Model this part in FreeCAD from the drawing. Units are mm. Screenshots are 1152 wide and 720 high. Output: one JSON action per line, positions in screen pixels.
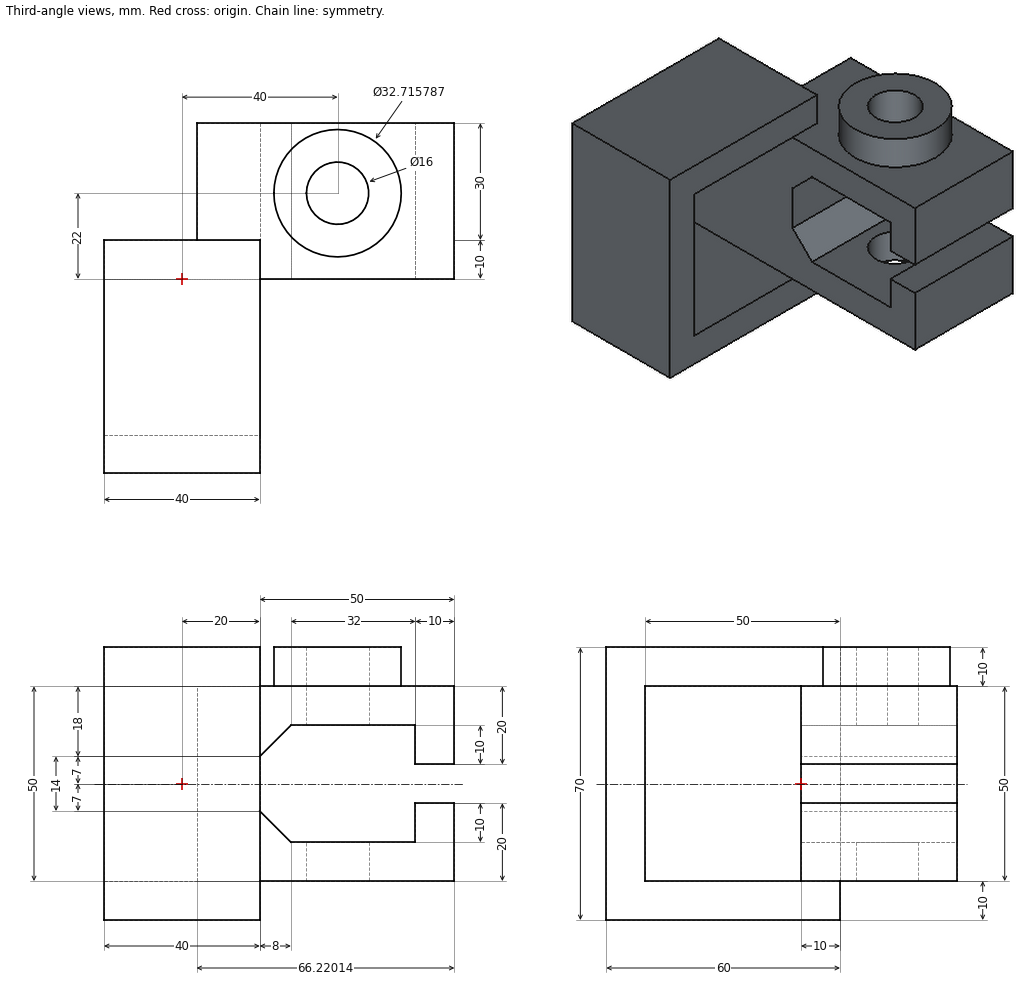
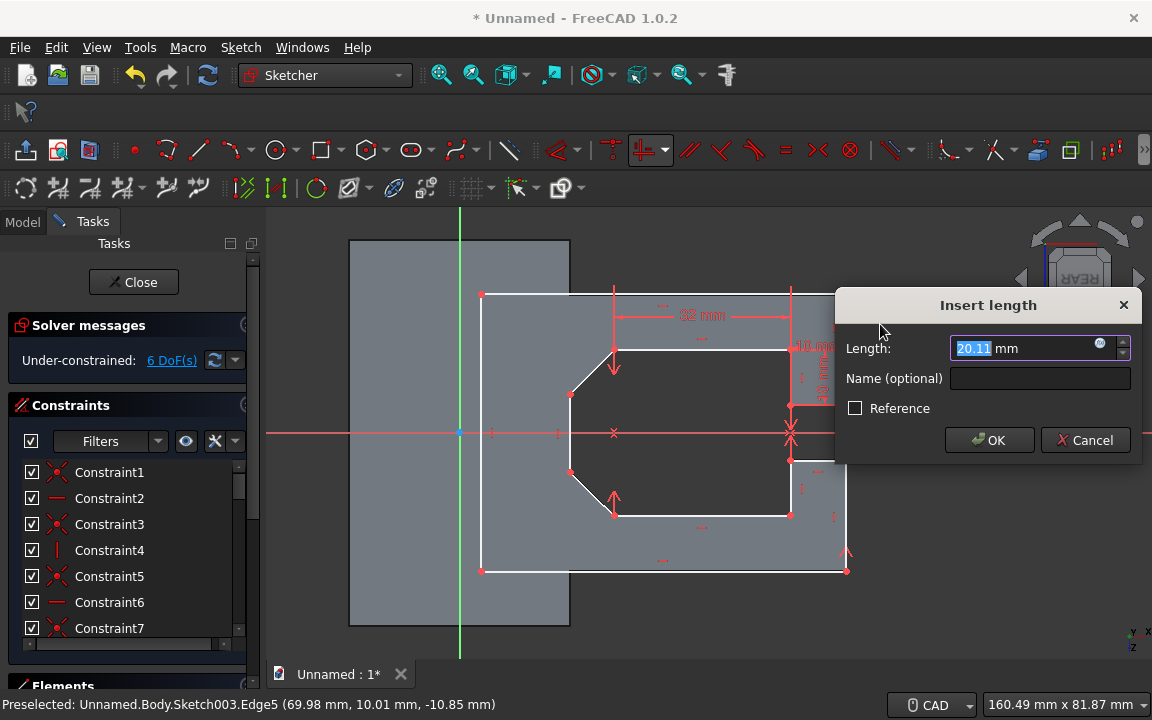
{"action": "type", "text": "20"}
{"action": "key", "text": "Return"}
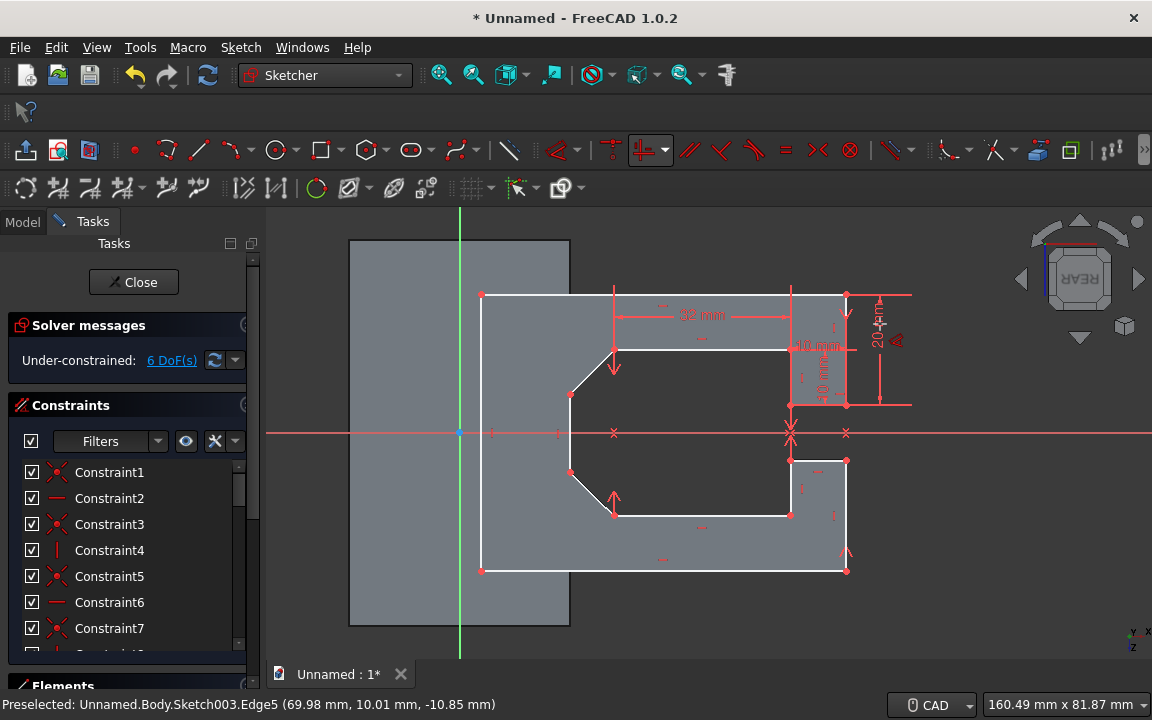
{"action": "left_click", "coordinate": [481, 378]}
{"action": "left_click", "coordinate": [515, 369]}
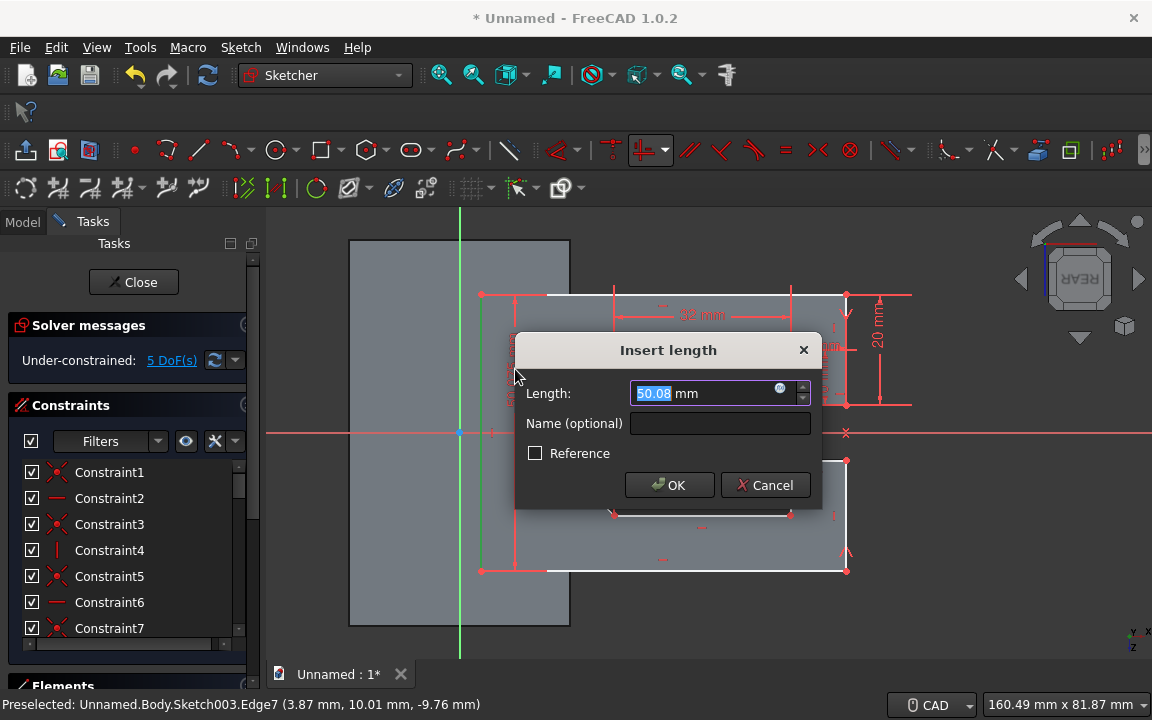
{"action": "type", "text": "50"}
{"action": "key", "text": "Return"}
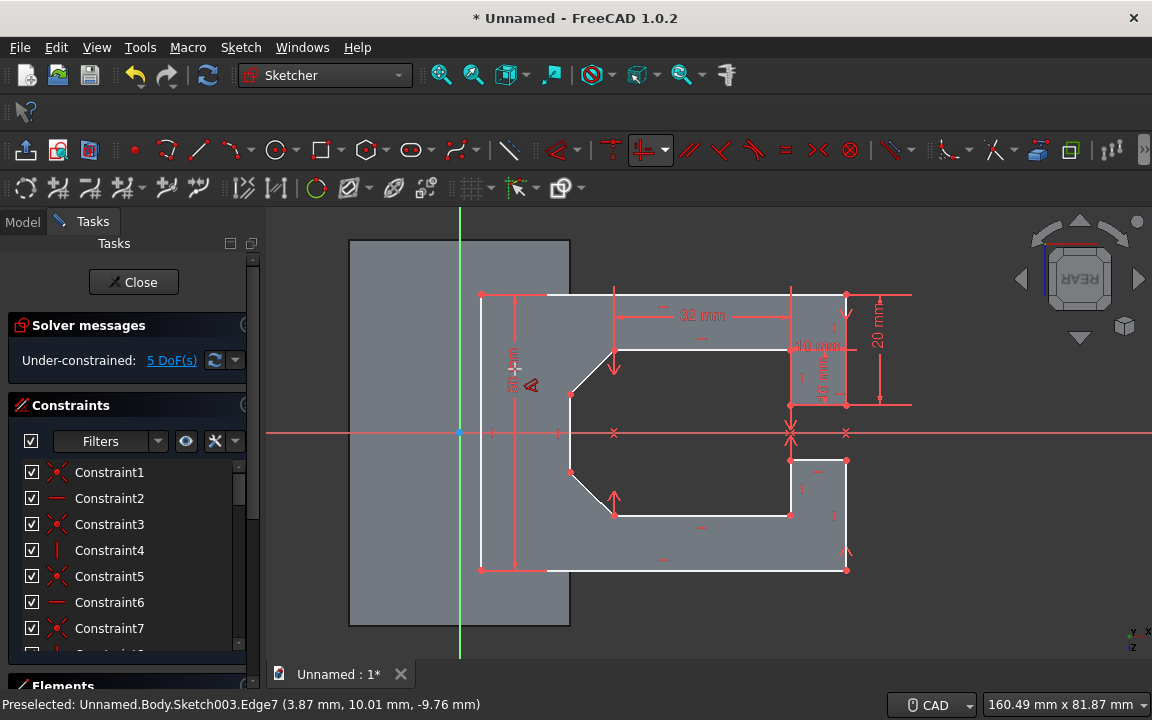
{"action": "left_click", "coordinate": [570, 450]}
{"action": "left_click", "coordinate": [536, 416]}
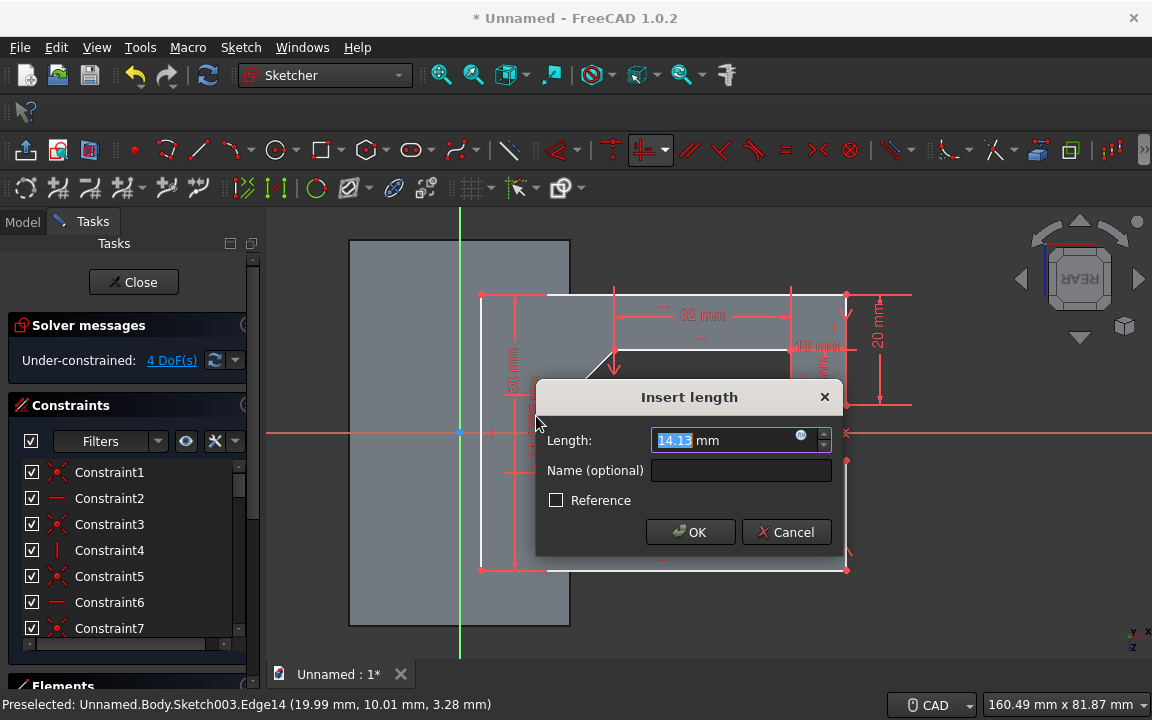
{"action": "type", "text": "14"}
{"action": "key", "text": "Return"}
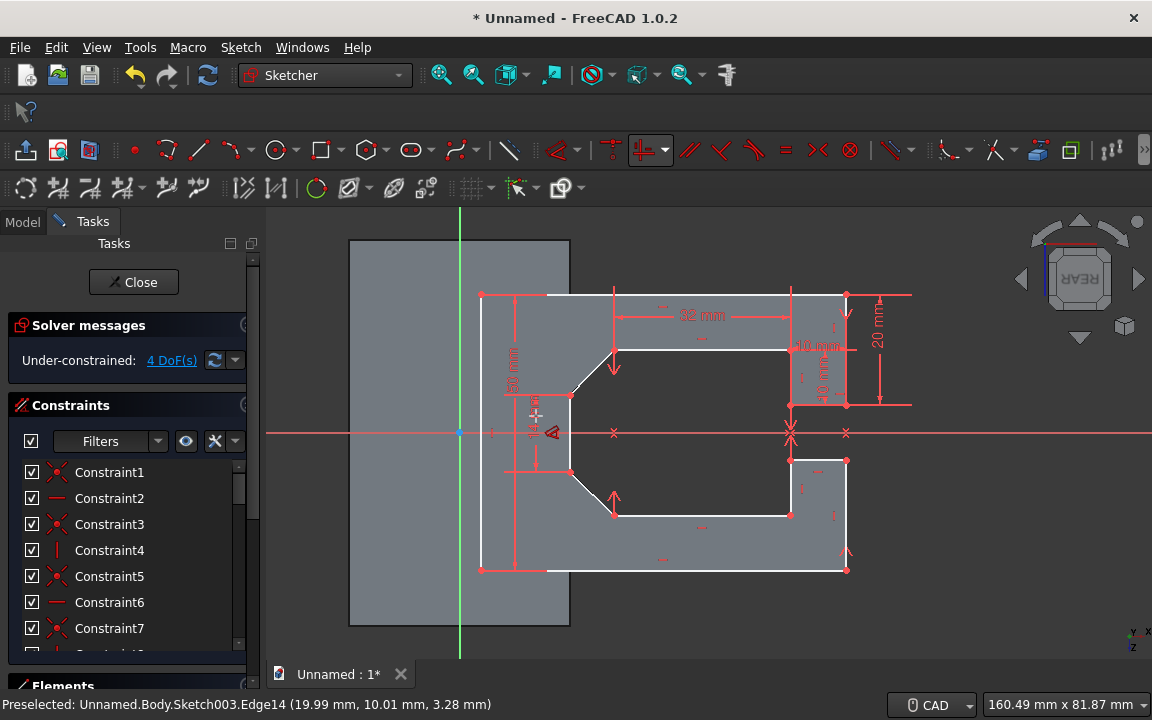
{"action": "left_click", "coordinate": [570, 395]}
{"action": "left_click", "coordinate": [426, 414]}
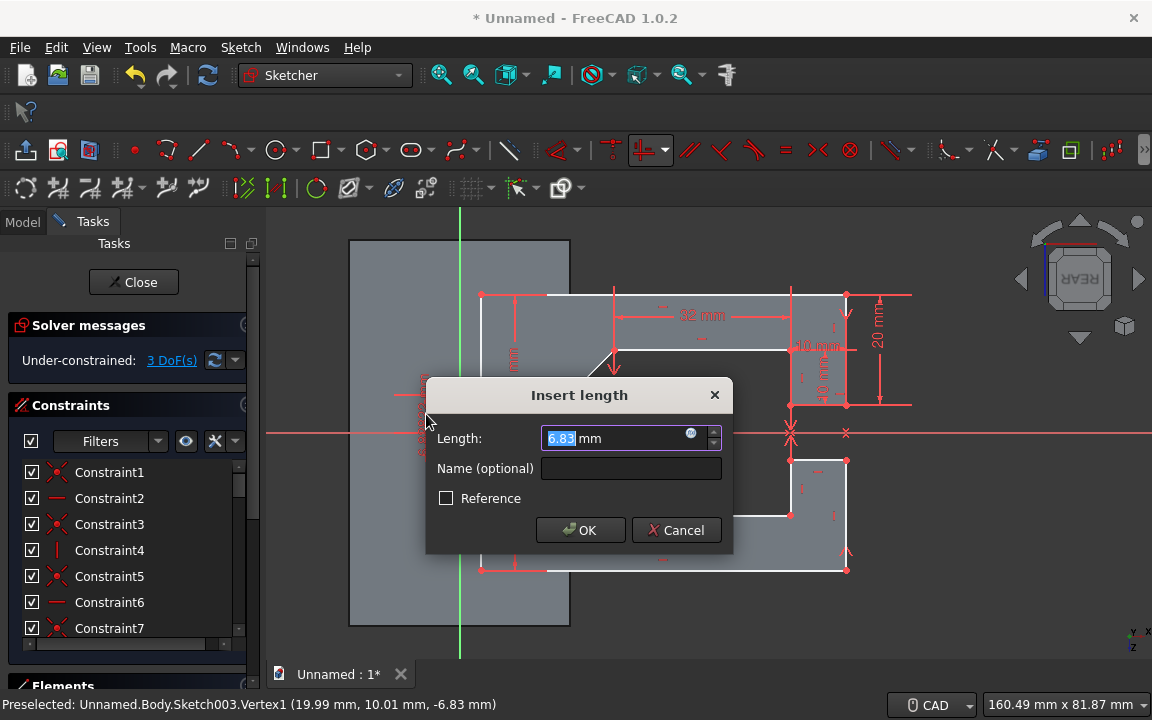
{"action": "type", "text": "7"}
{"action": "key", "text": "Return"}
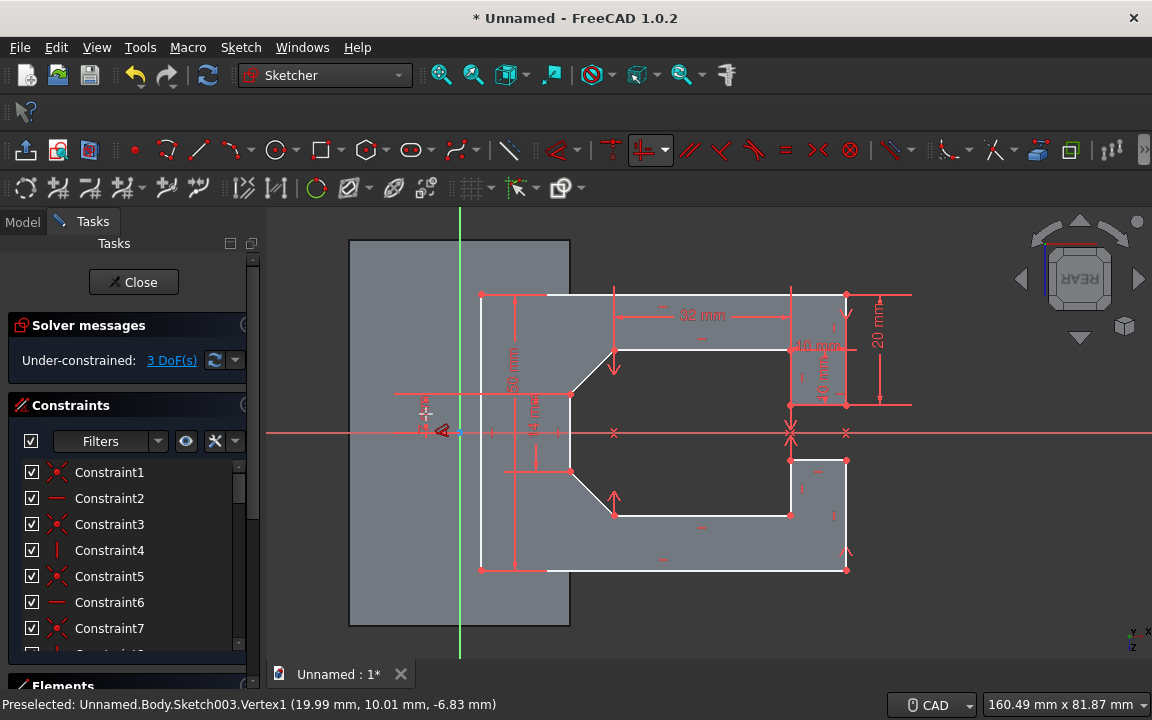
{"action": "left_click", "coordinate": [583, 381]}
{"action": "left_click", "coordinate": [592, 316]}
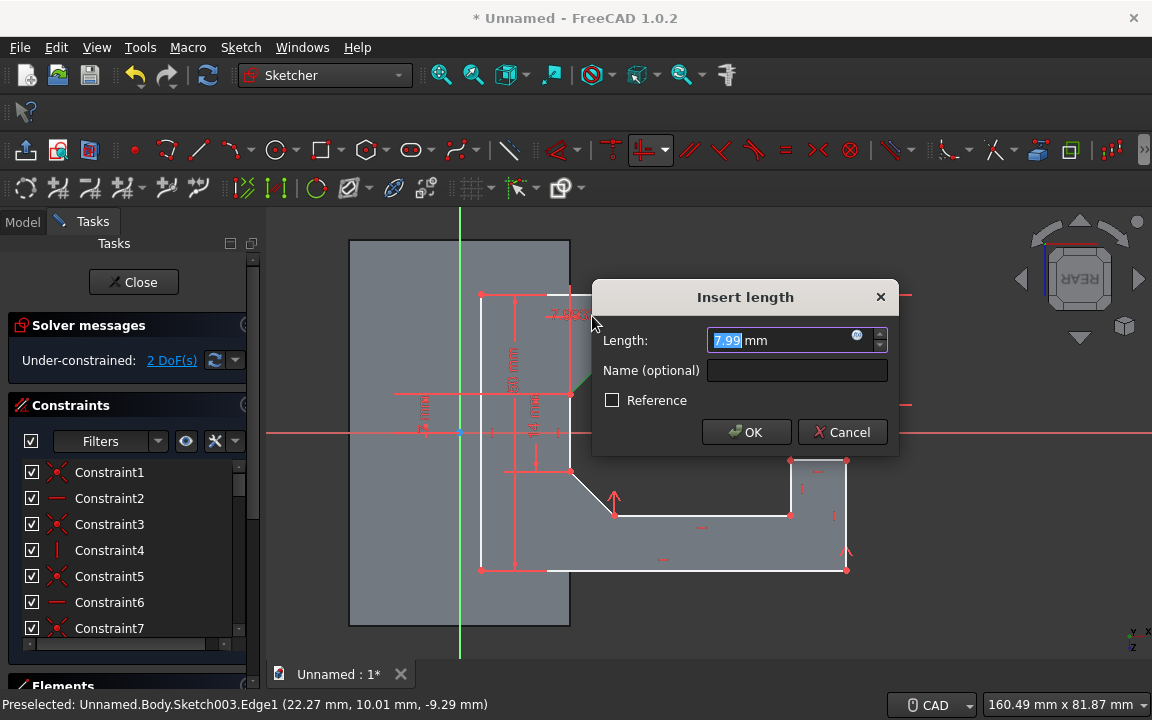
{"action": "type", "text": "8"}
{"action": "key", "text": "Return"}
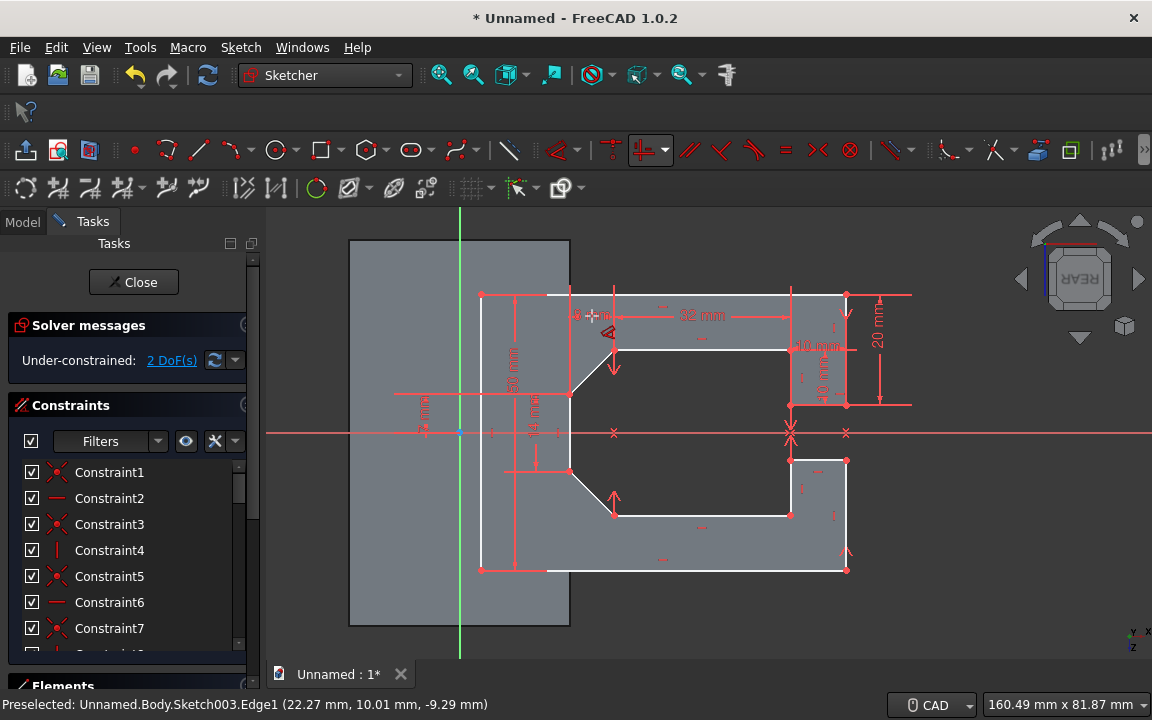
{"action": "left_click", "coordinate": [570, 394]}
{"action": "left_click", "coordinate": [515, 467]}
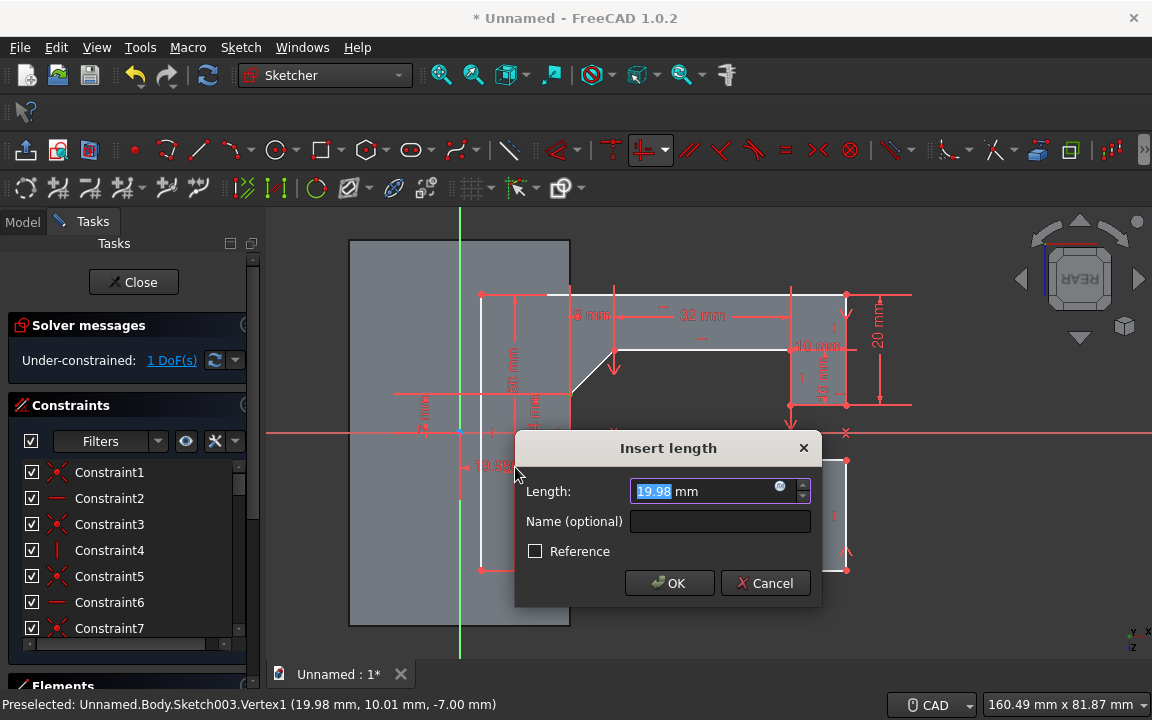
{"action": "type", "text": "20"}
{"action": "key", "text": "Return"}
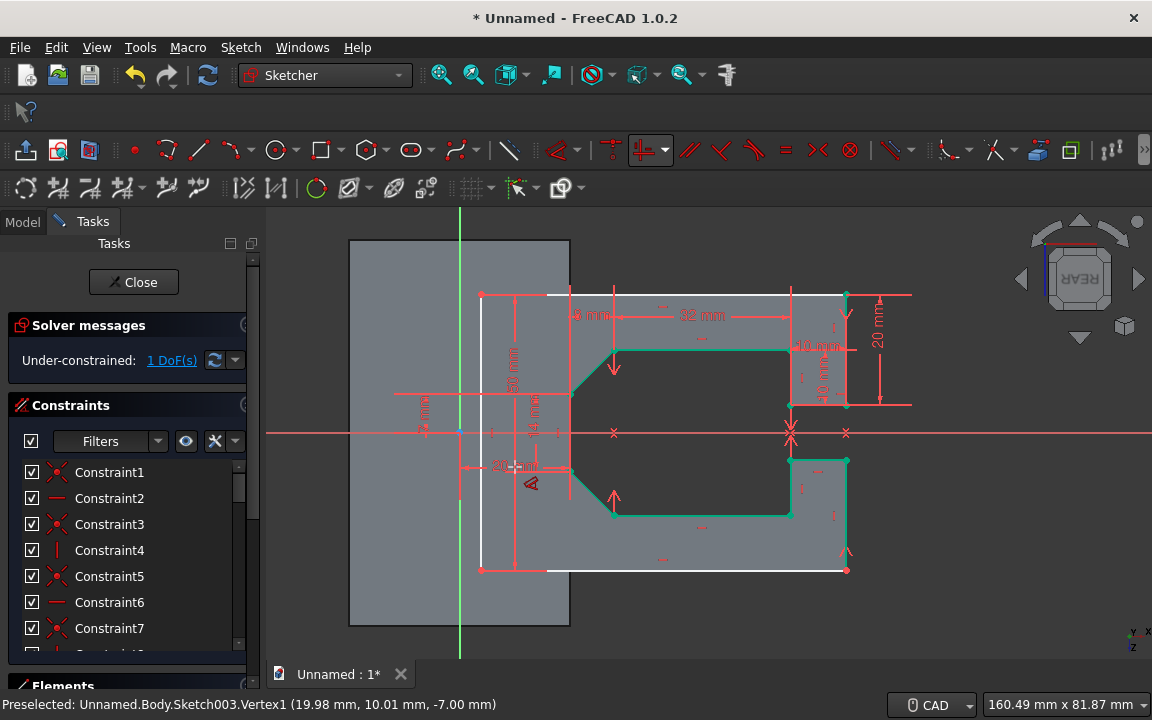
{"action": "left_click", "coordinate": [737, 295]}
{"action": "left_click", "coordinate": [664, 261]}